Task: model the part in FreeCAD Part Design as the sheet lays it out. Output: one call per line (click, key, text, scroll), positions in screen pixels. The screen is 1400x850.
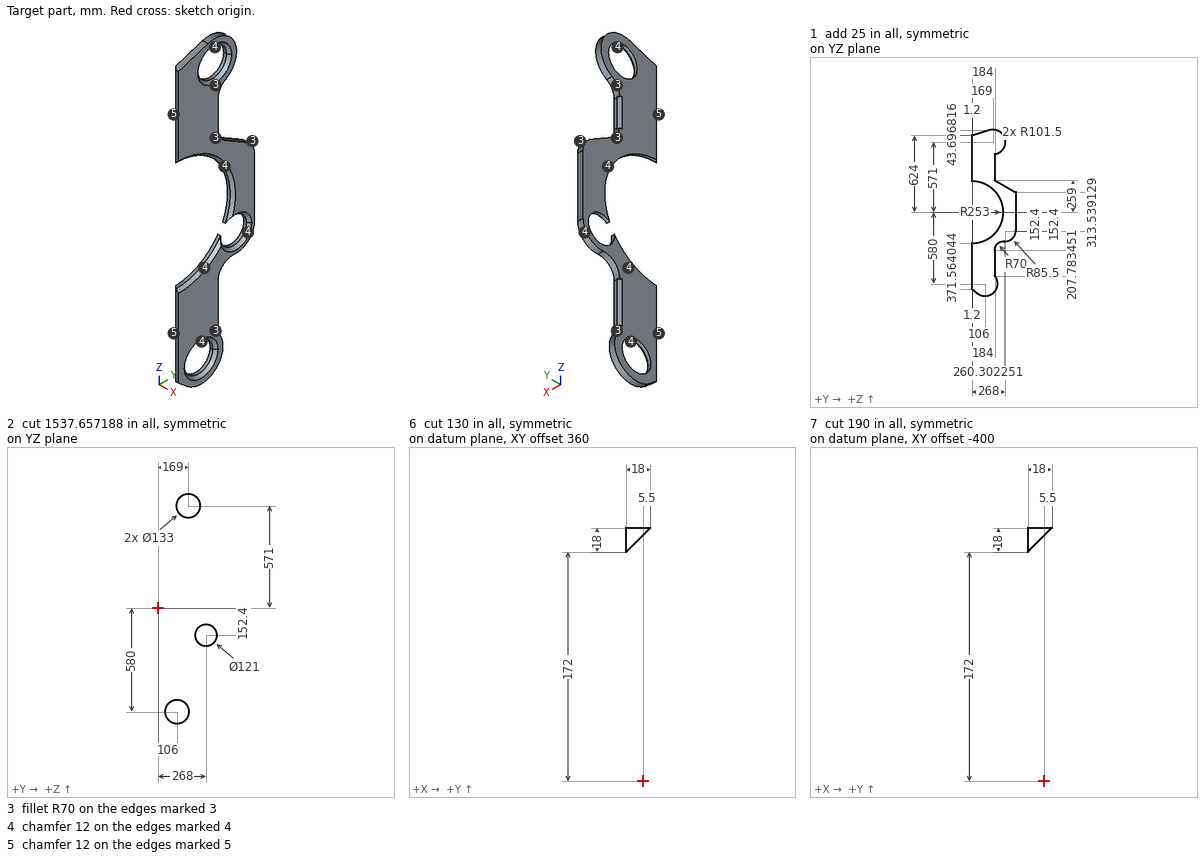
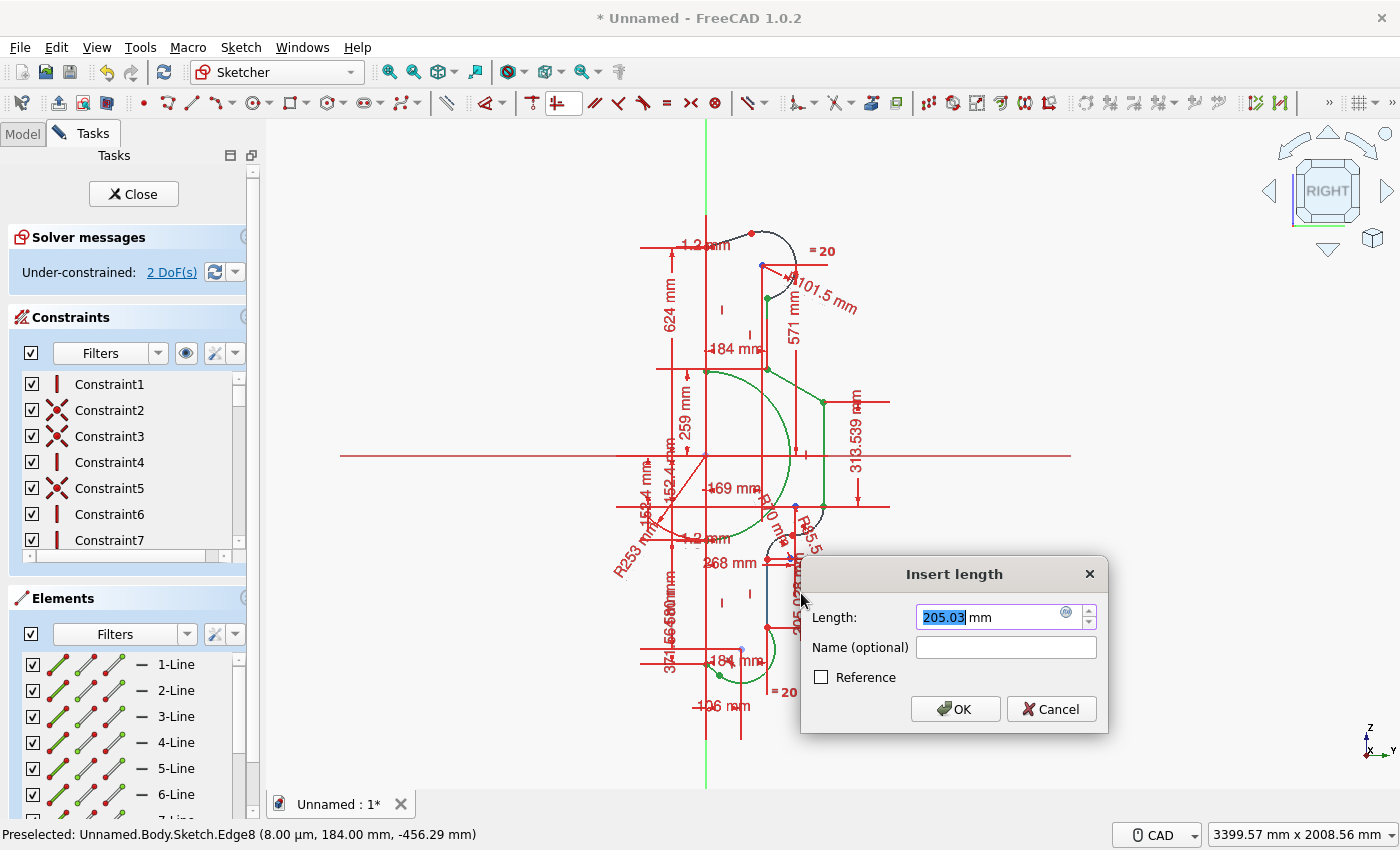
text(207.783451)
key(Return)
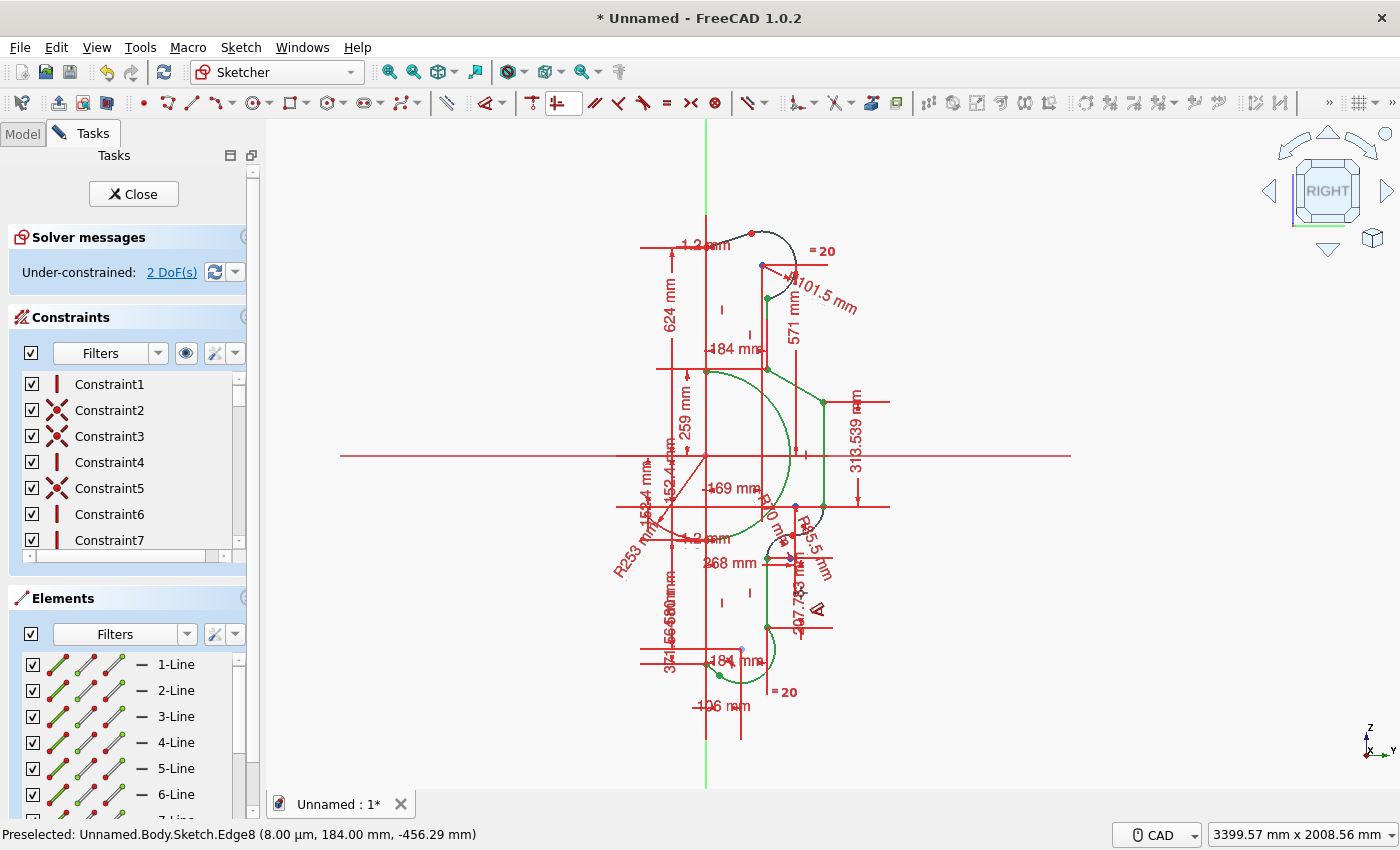
scroll(738, 237, up, 6)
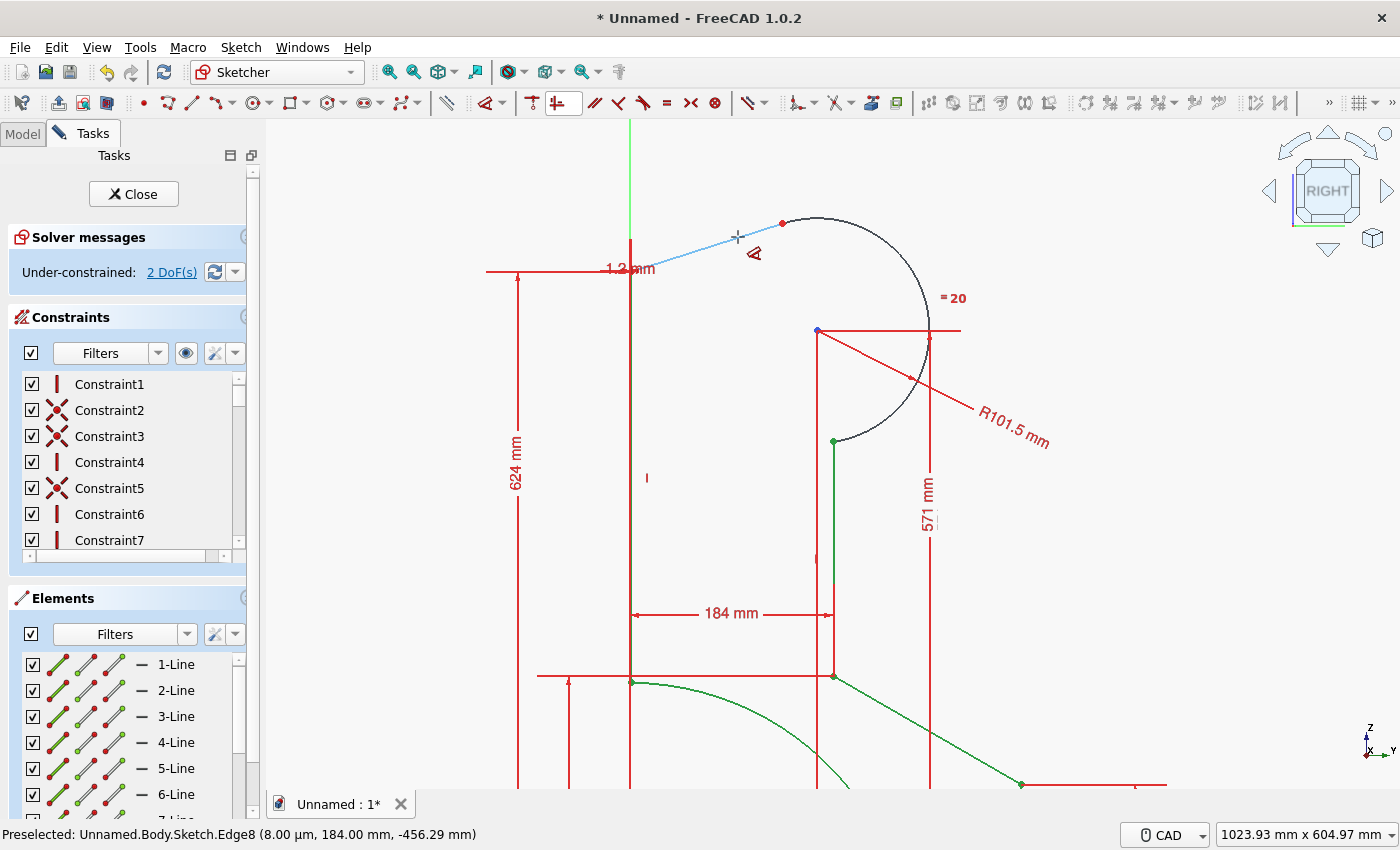
click(737, 238)
click(597, 248)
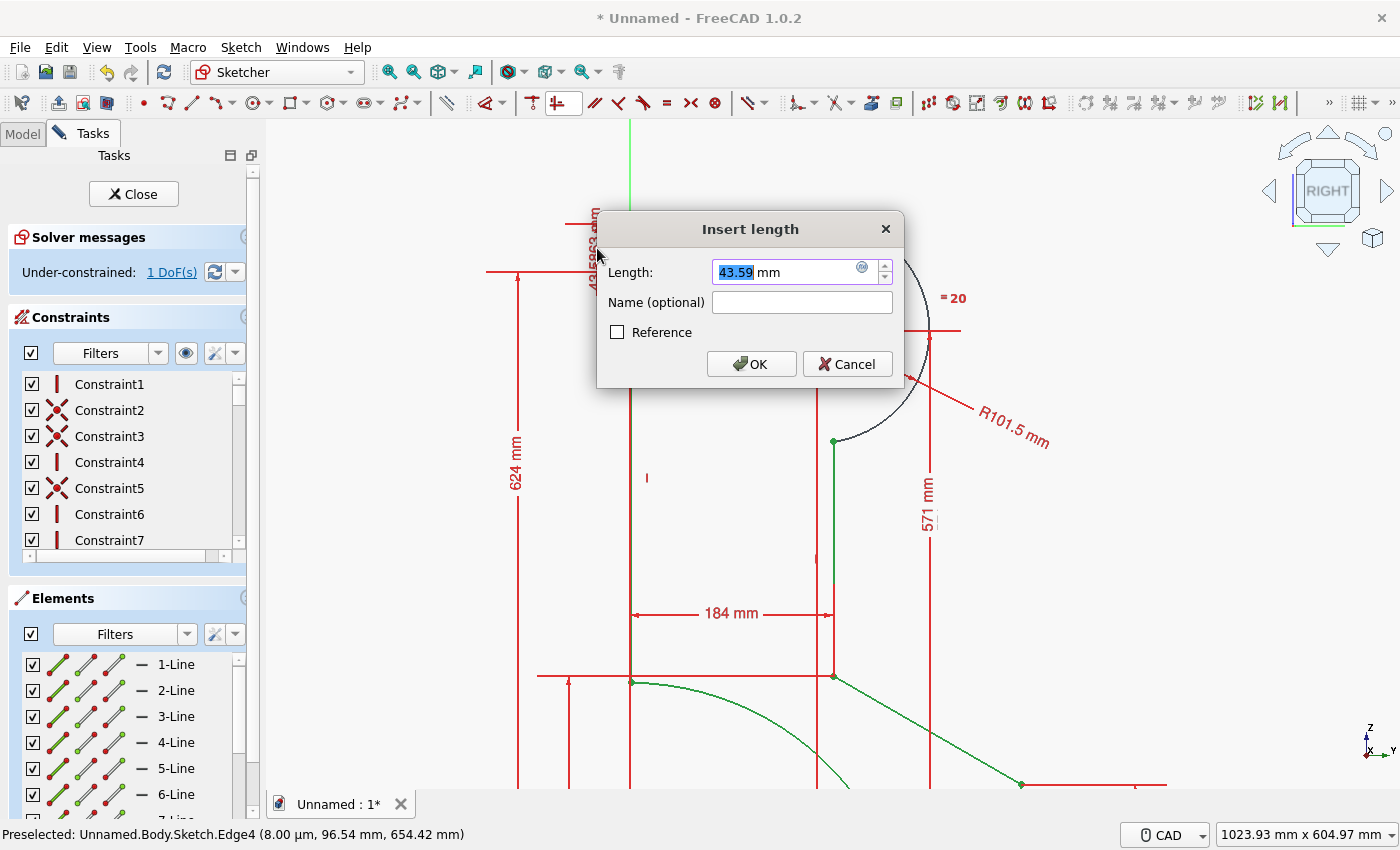
text(43.696816)
key(Return)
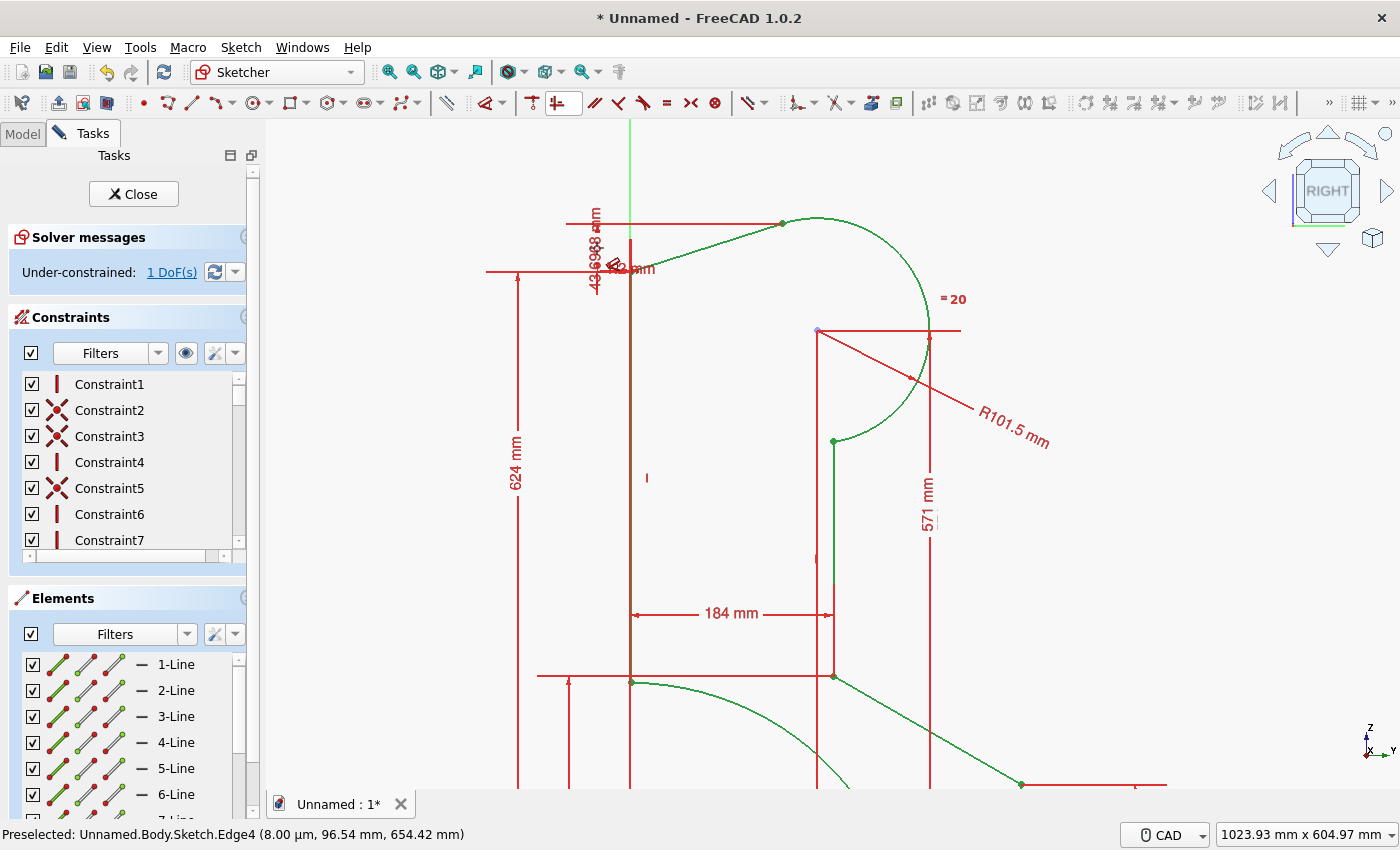
scroll(738, 237, down, 6)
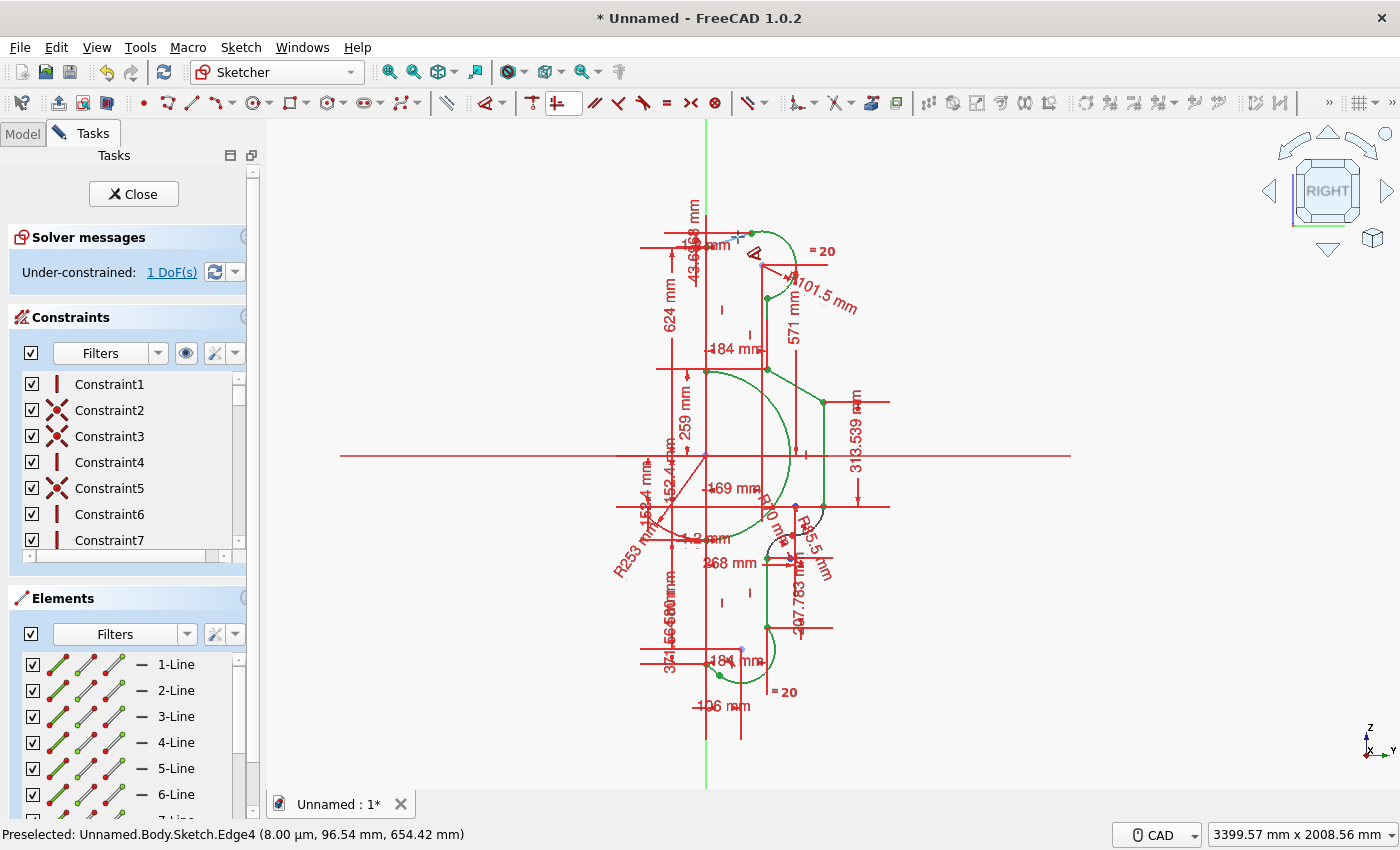
click(792, 535)
click(749, 617)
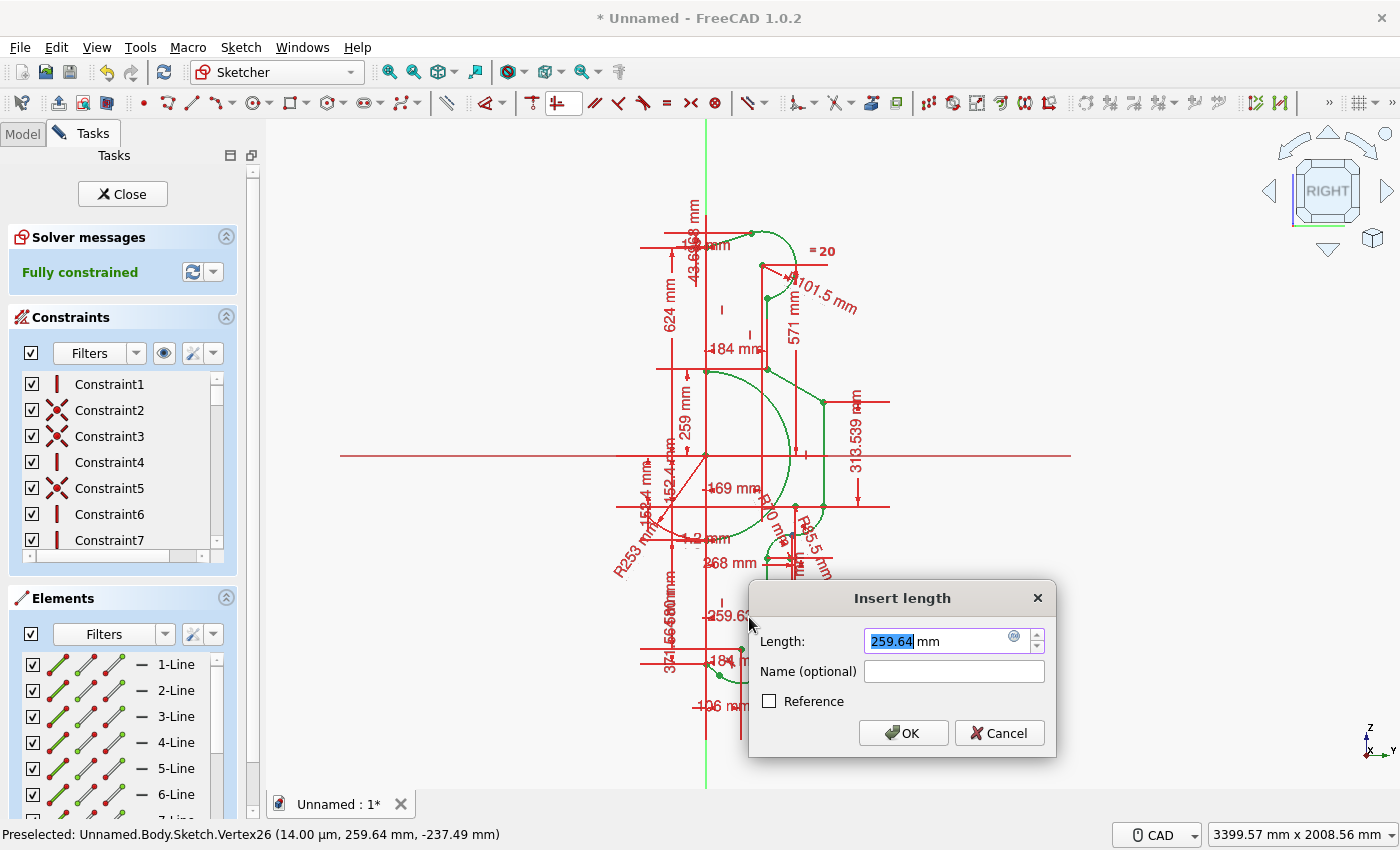
text(260.302251)
key(Return)
key(Escape)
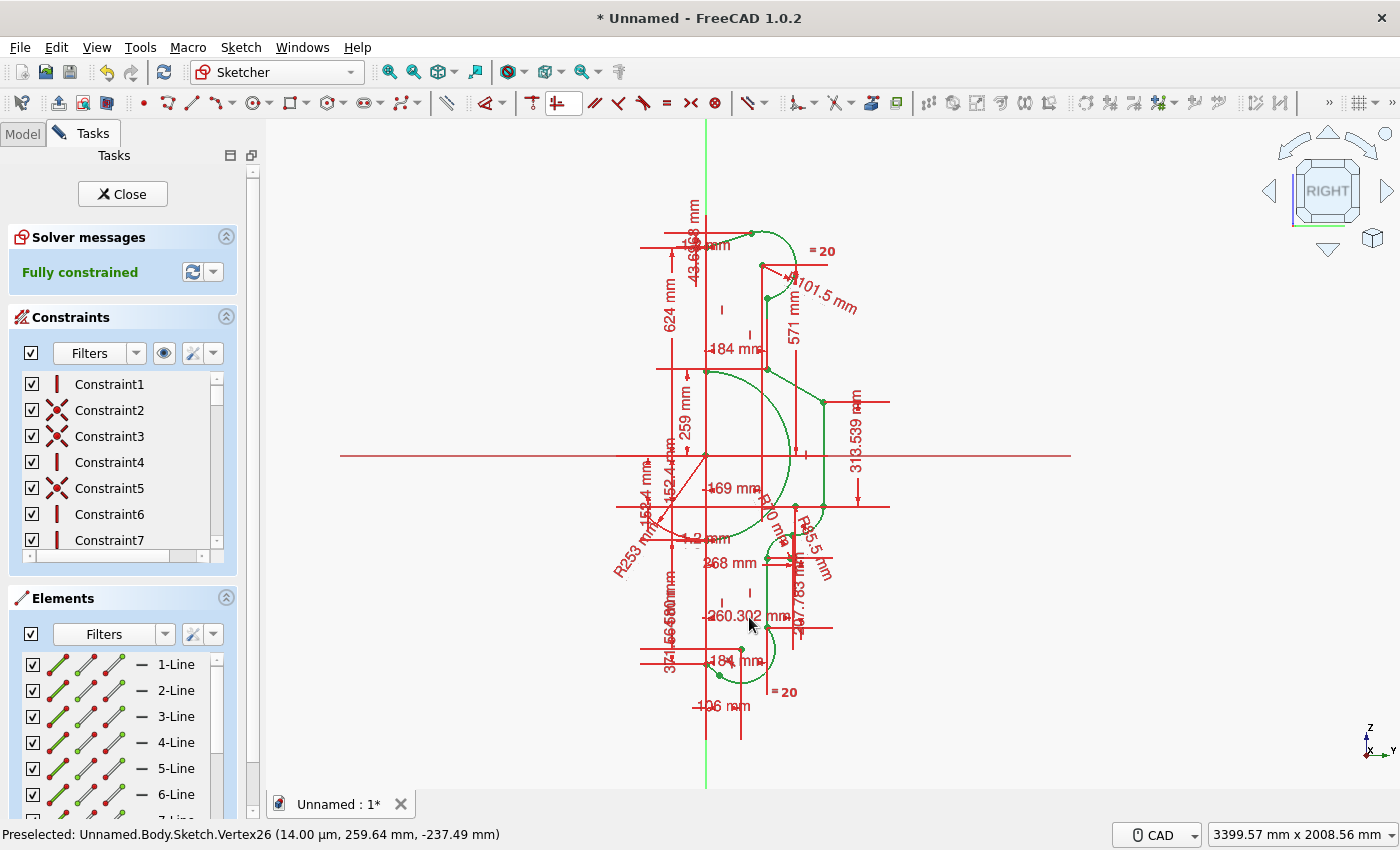
click(123, 194)